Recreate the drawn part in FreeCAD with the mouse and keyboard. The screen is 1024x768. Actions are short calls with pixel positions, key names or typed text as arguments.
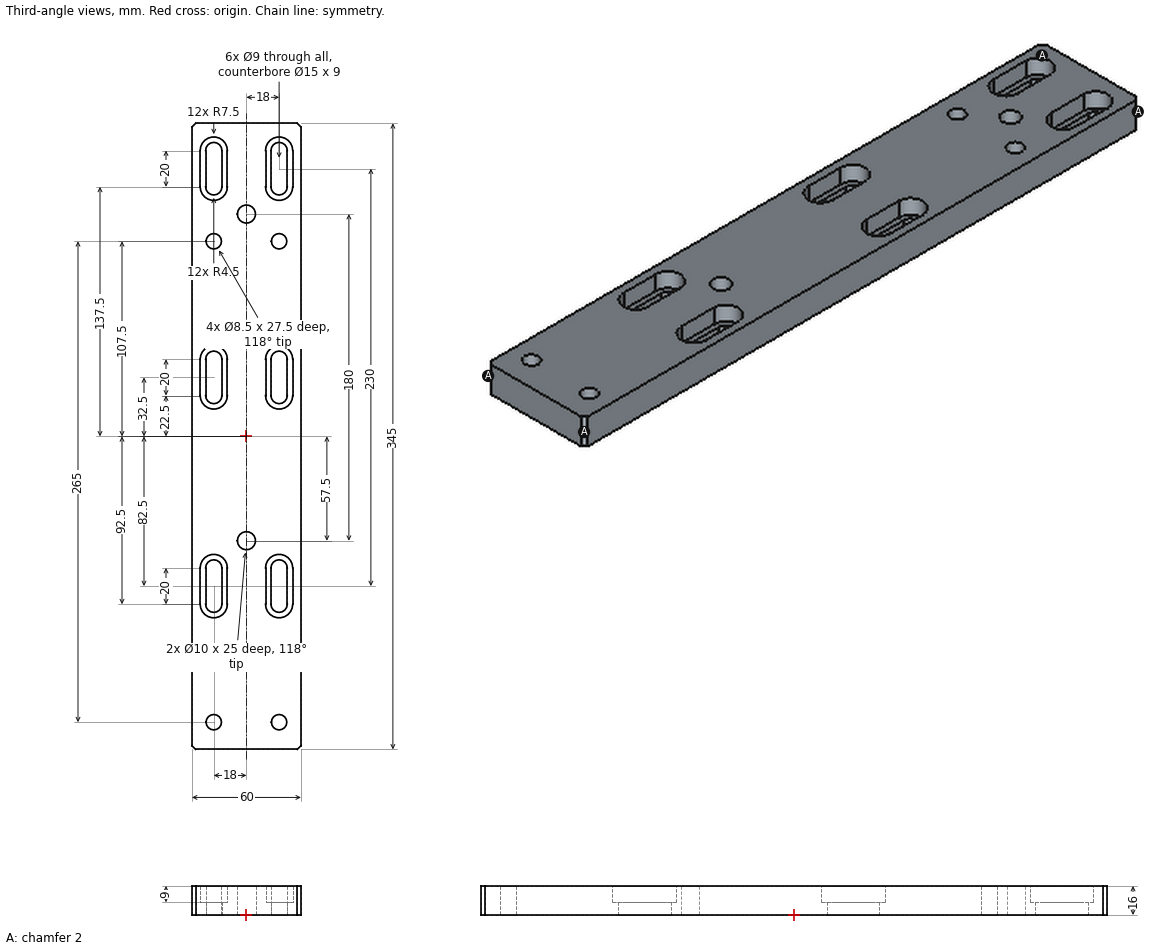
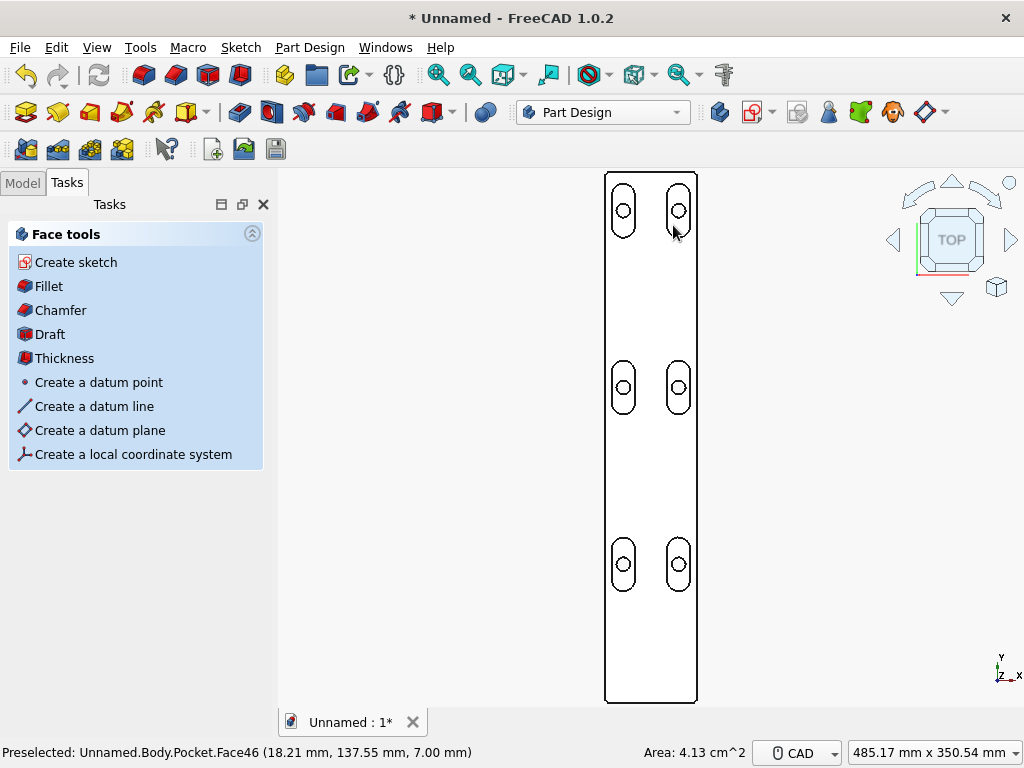
click(752, 112)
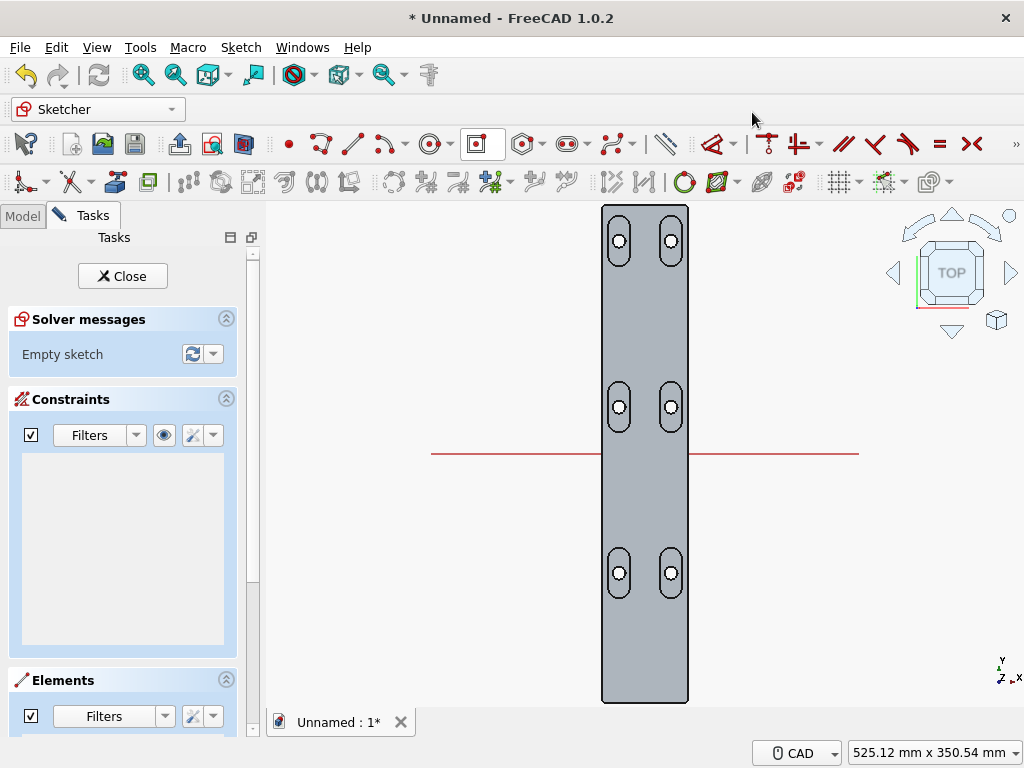
key(q)
key(s)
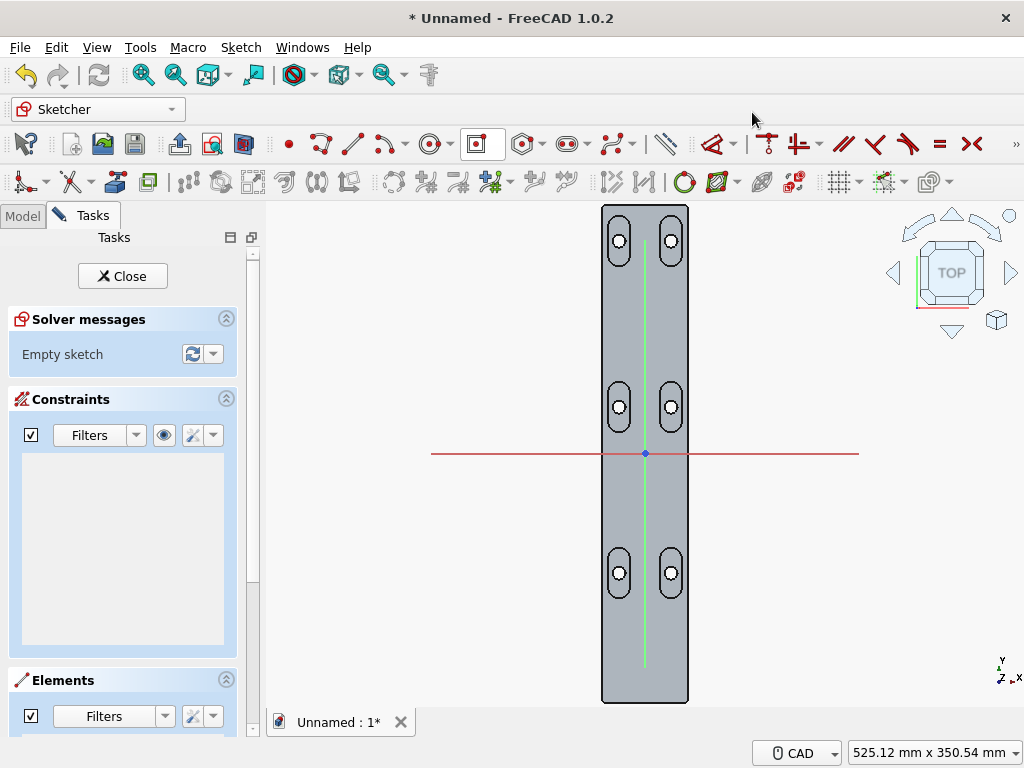
scroll(294, 666, down, 1)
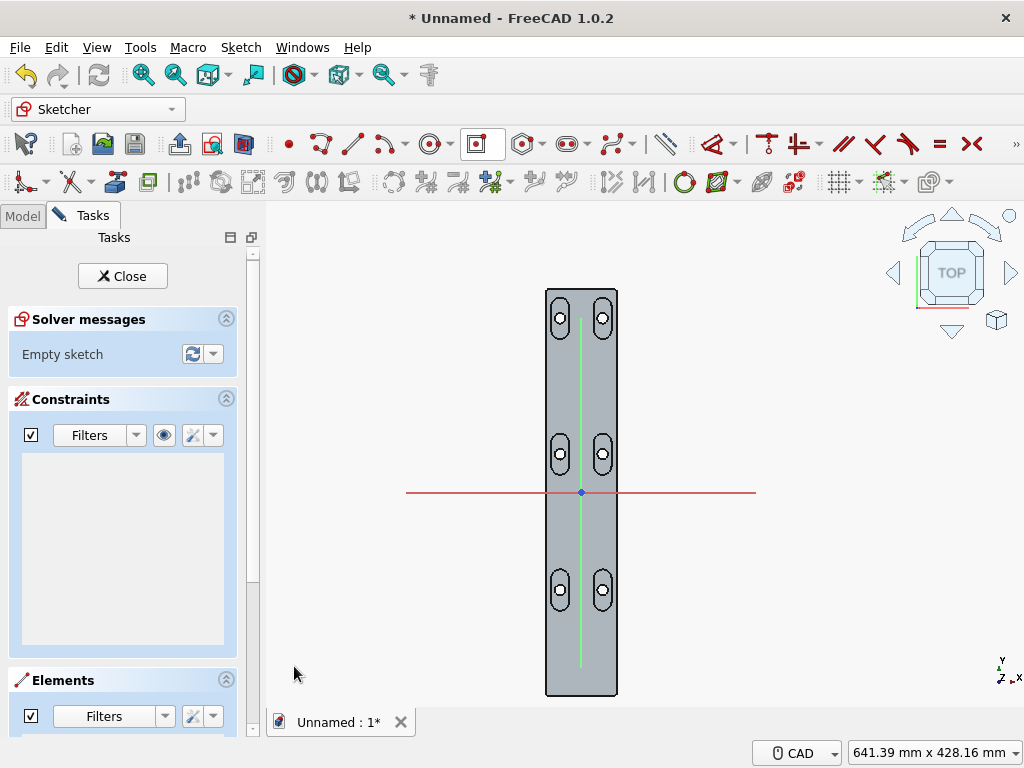
key(g)
key(s)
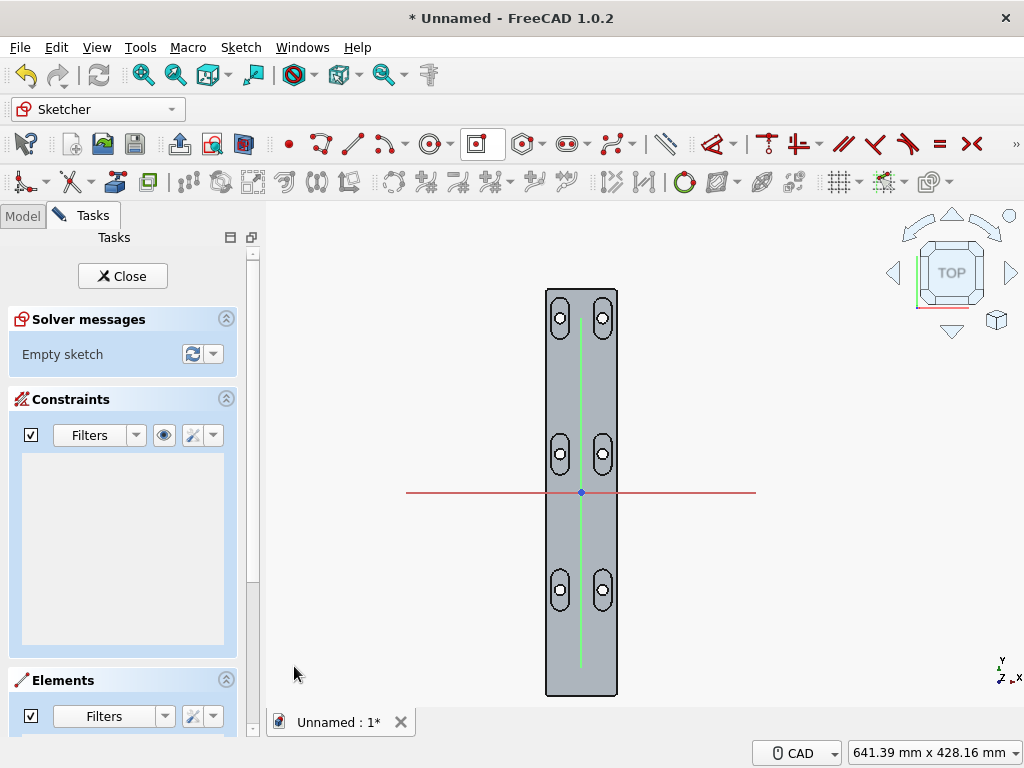
scroll(560, 330, up, 8)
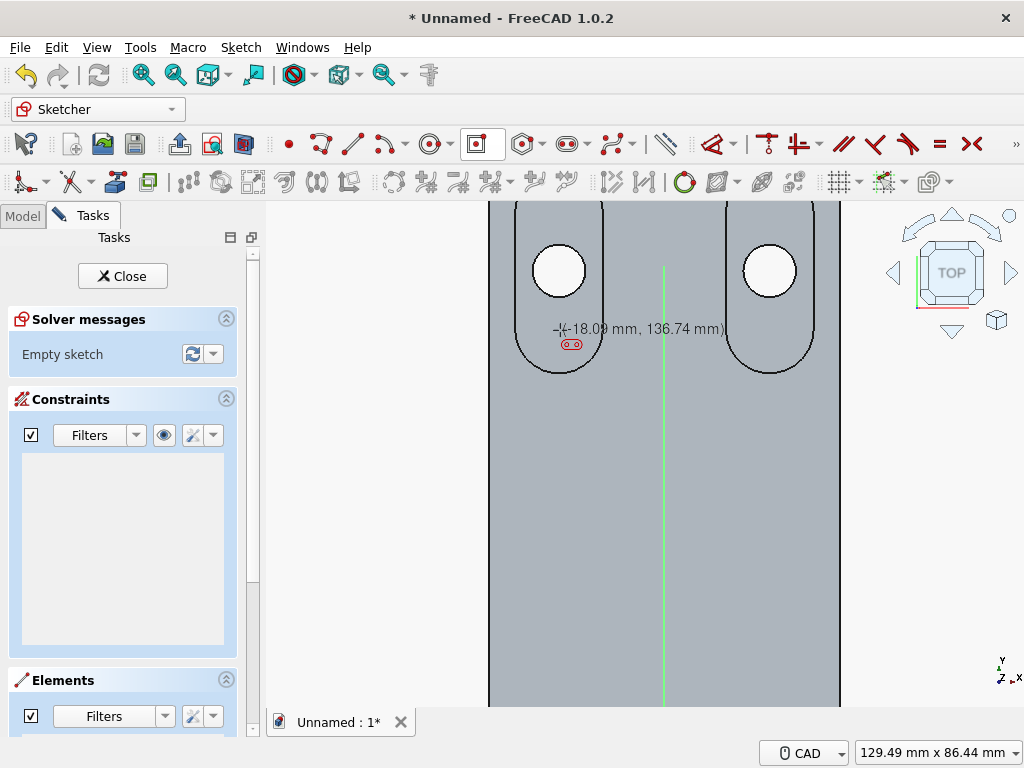
scroll(554, 330, down, 8)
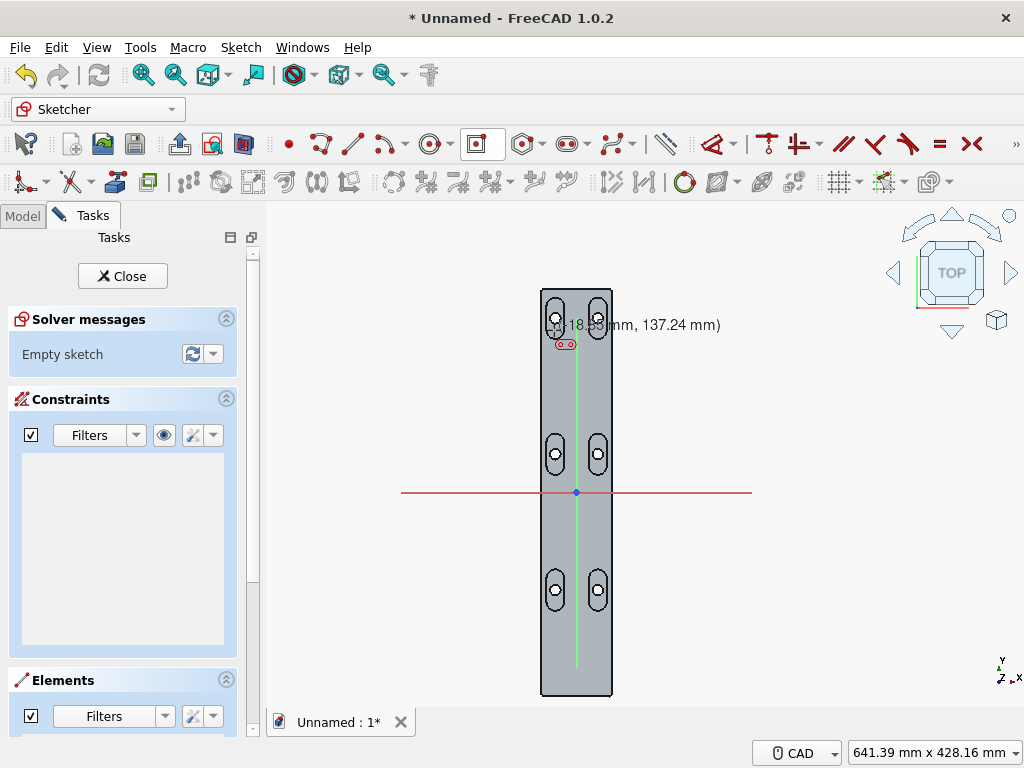
click(555, 330)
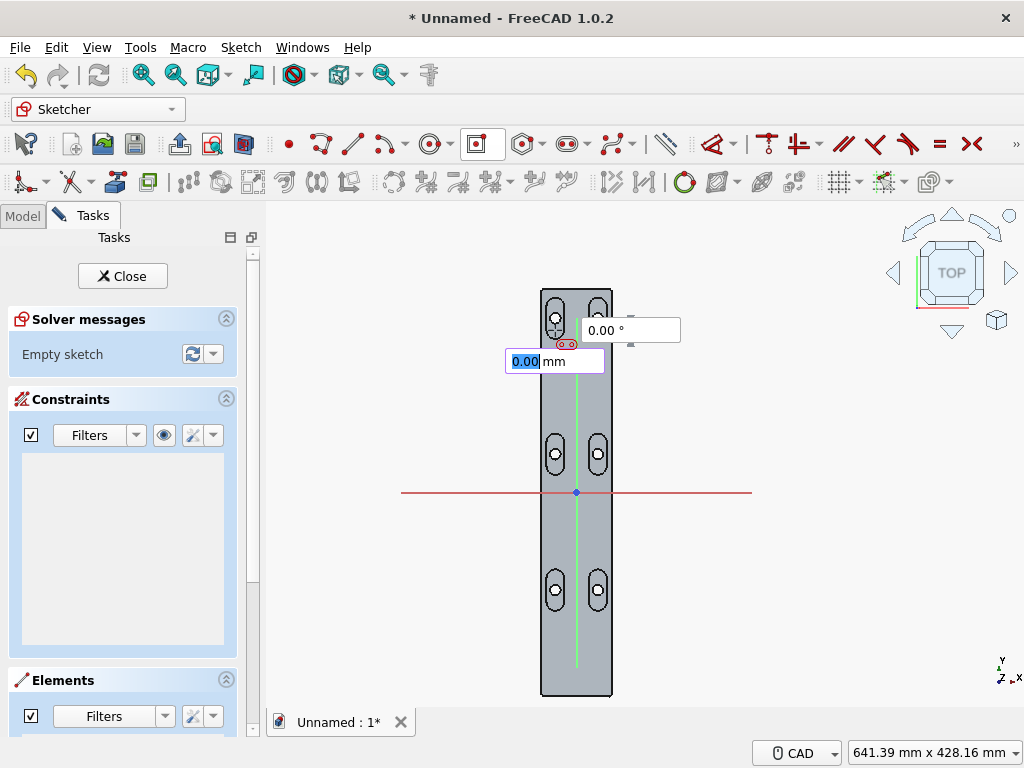
click(555, 306)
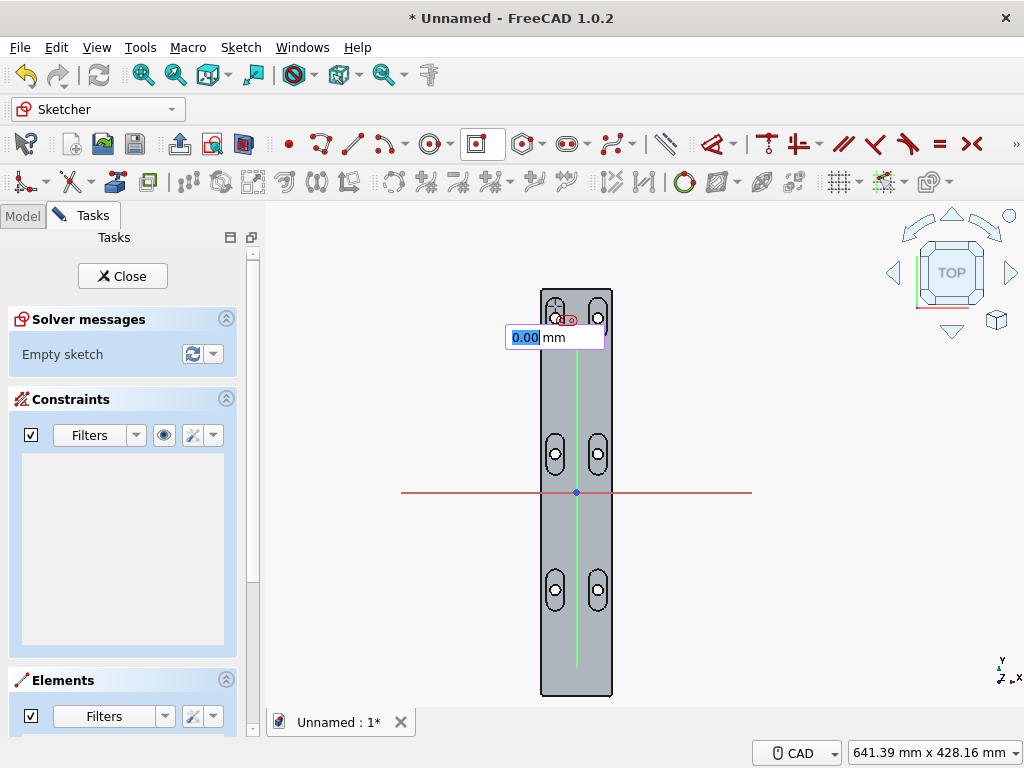
scroll(550, 318, up, 6)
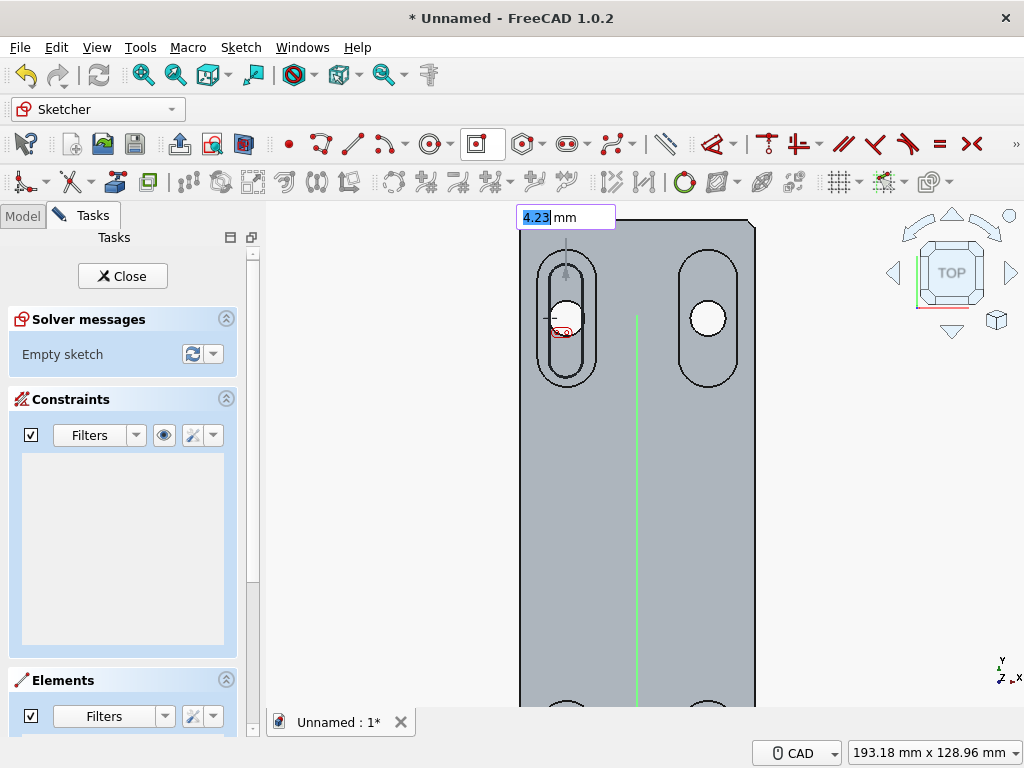
click(549, 318)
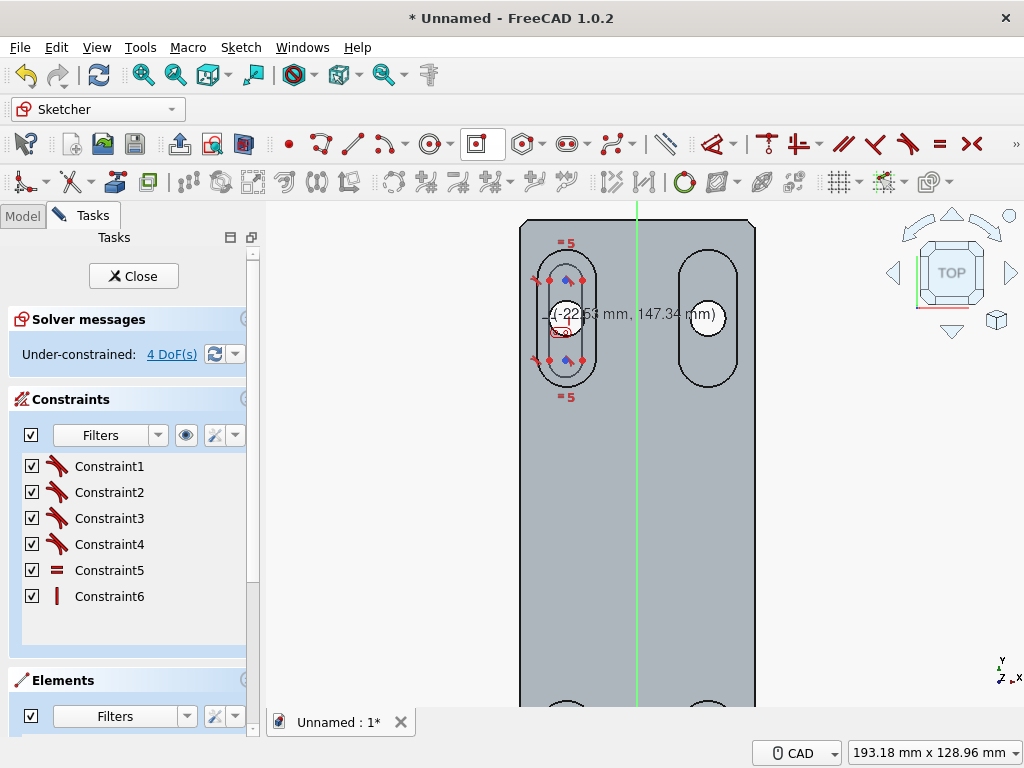
scroll(708, 358, up, 2)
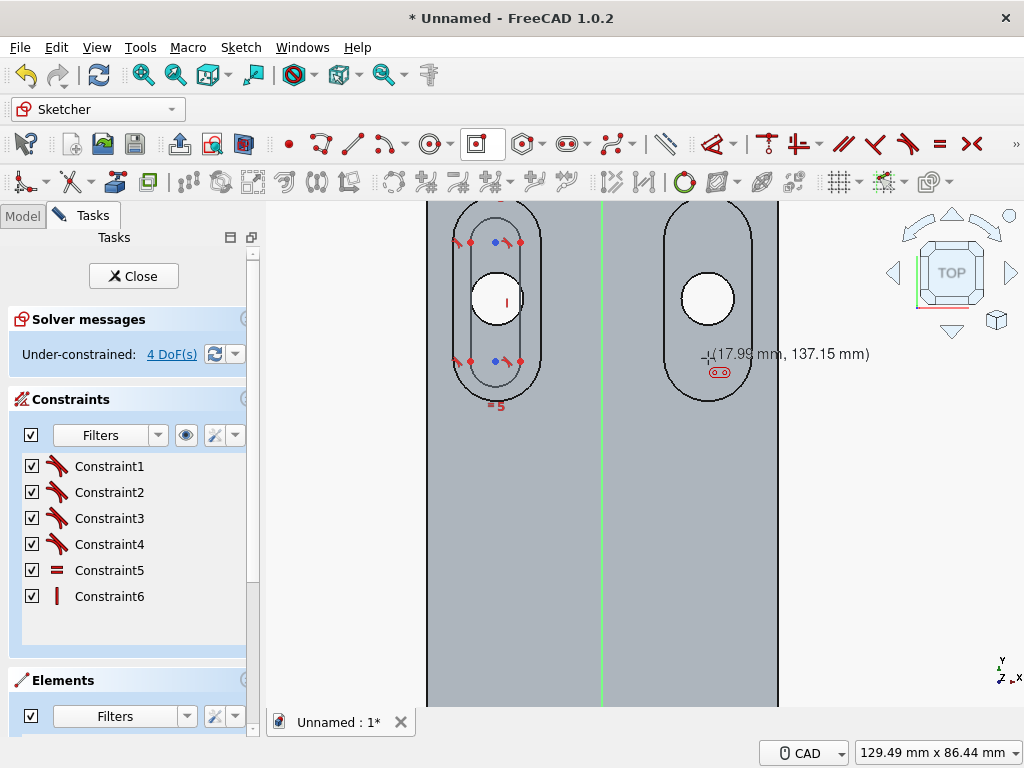
scroll(570, 323, down, 8)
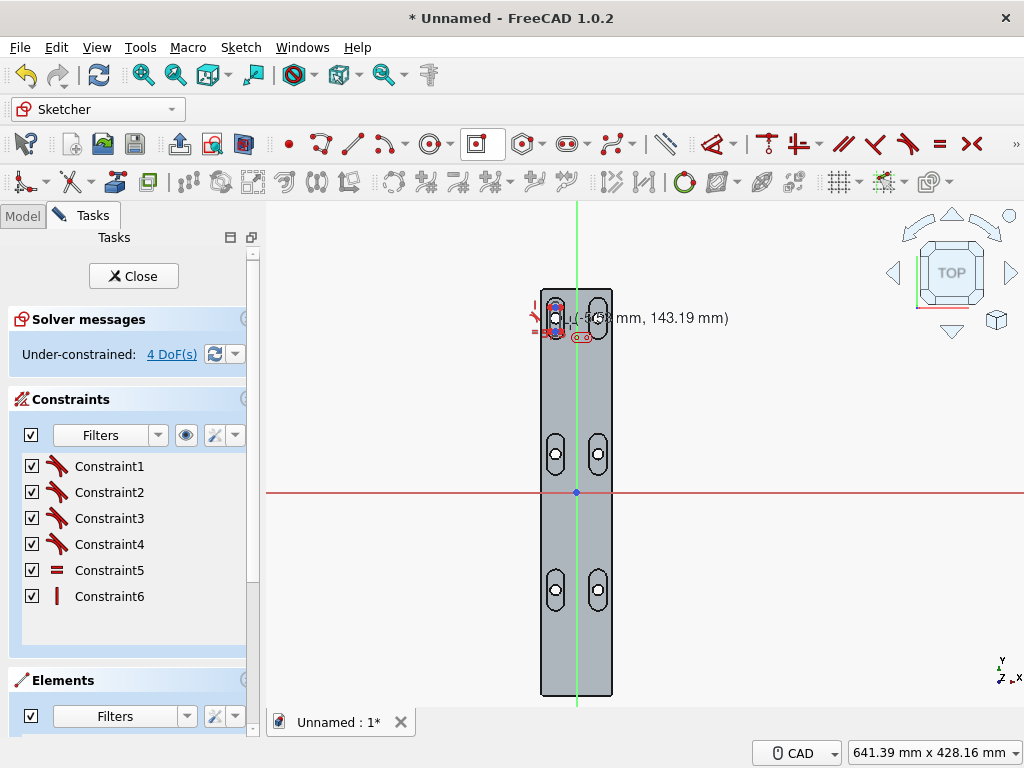
click(598, 330)